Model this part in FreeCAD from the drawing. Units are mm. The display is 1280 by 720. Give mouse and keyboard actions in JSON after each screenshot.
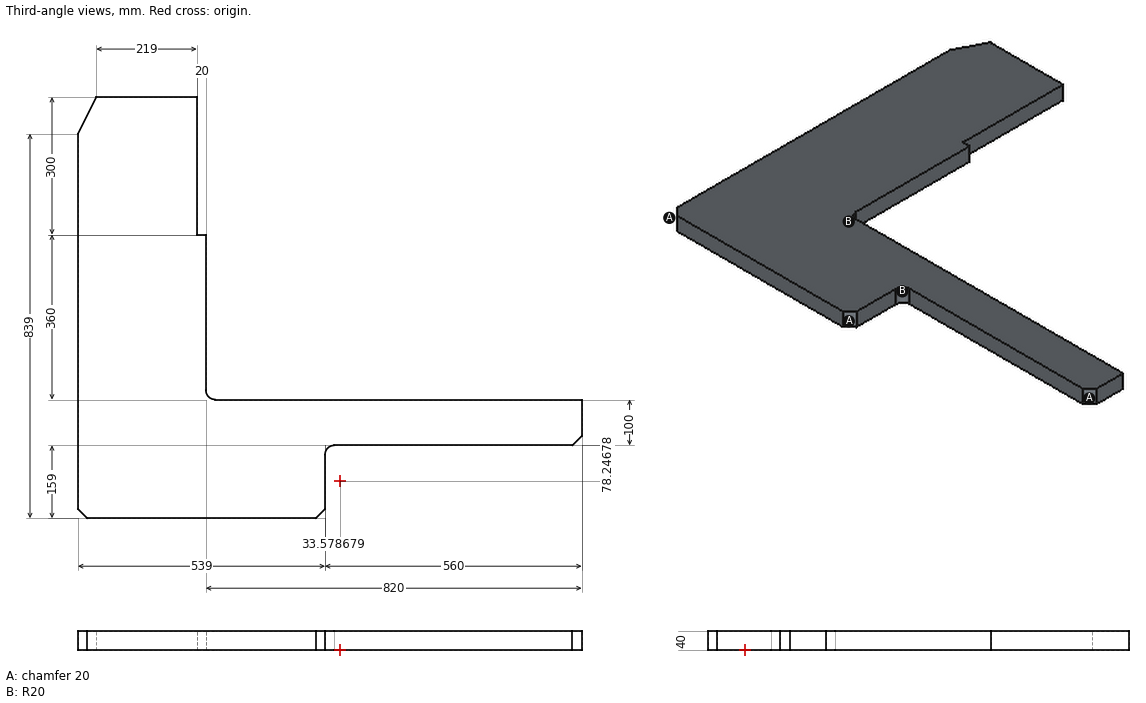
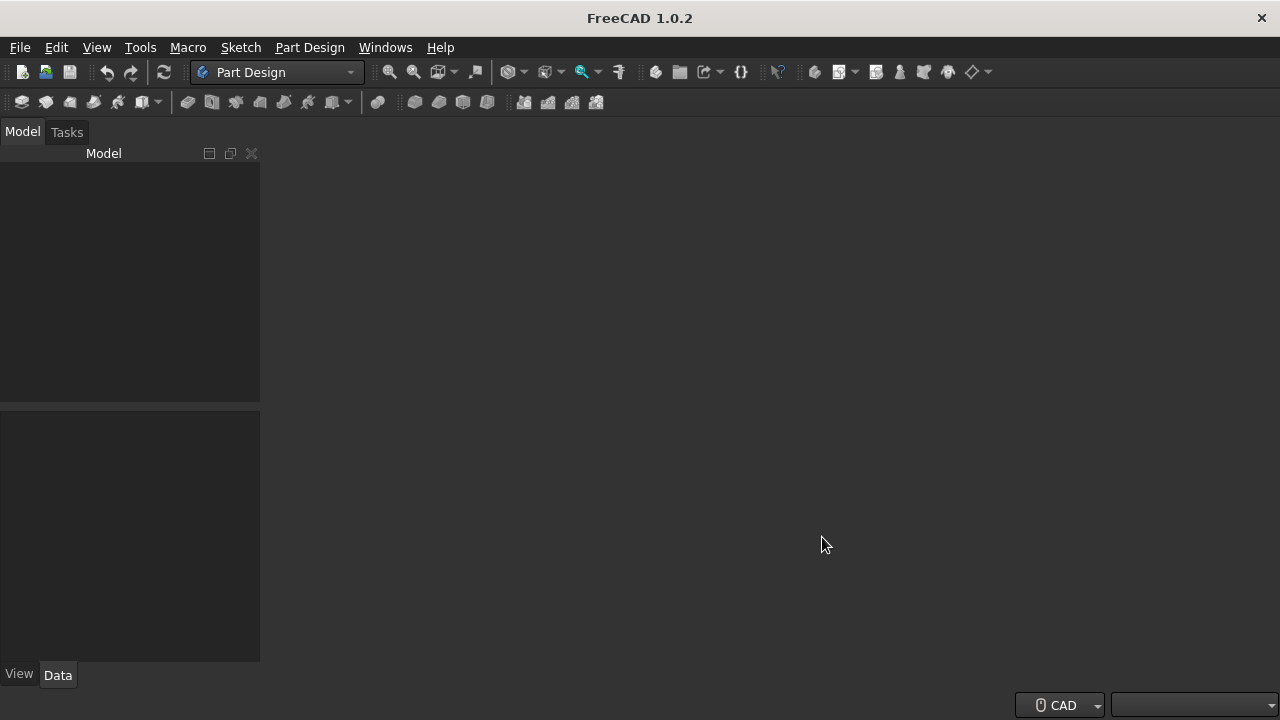
{"action": "key", "text": "ctrl+n"}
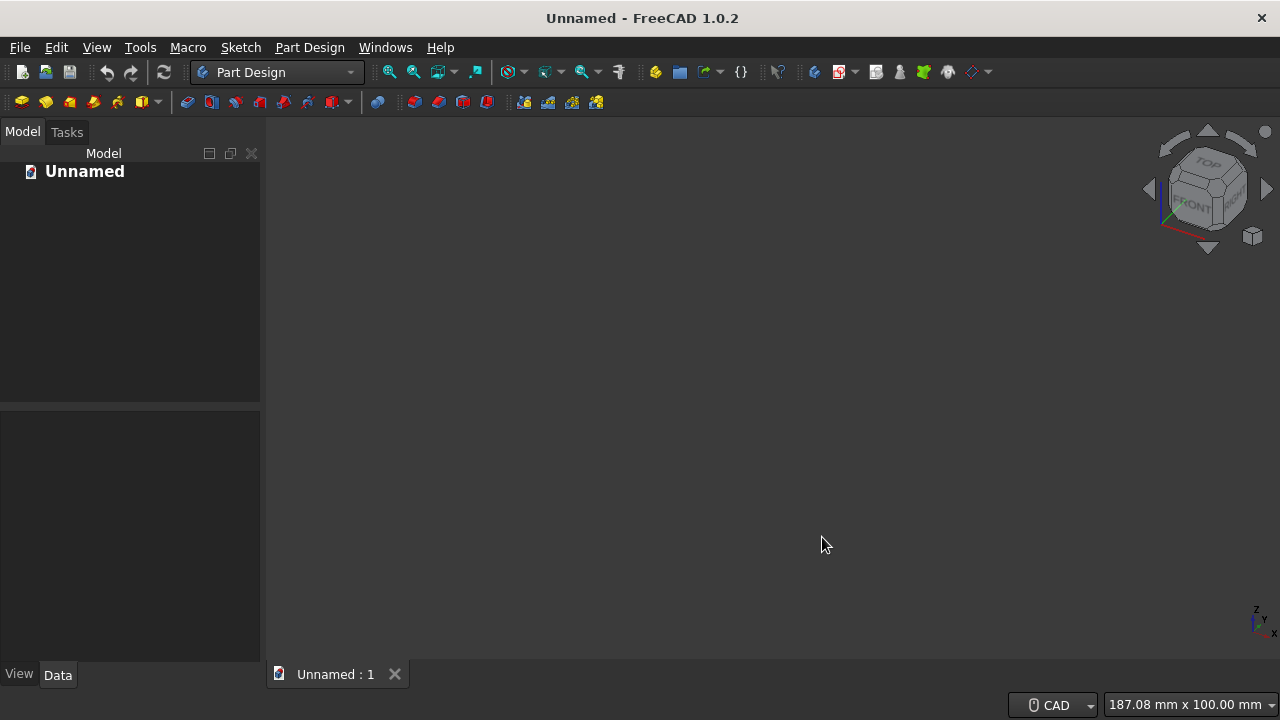
{"action": "left_click", "coordinate": [840, 72]}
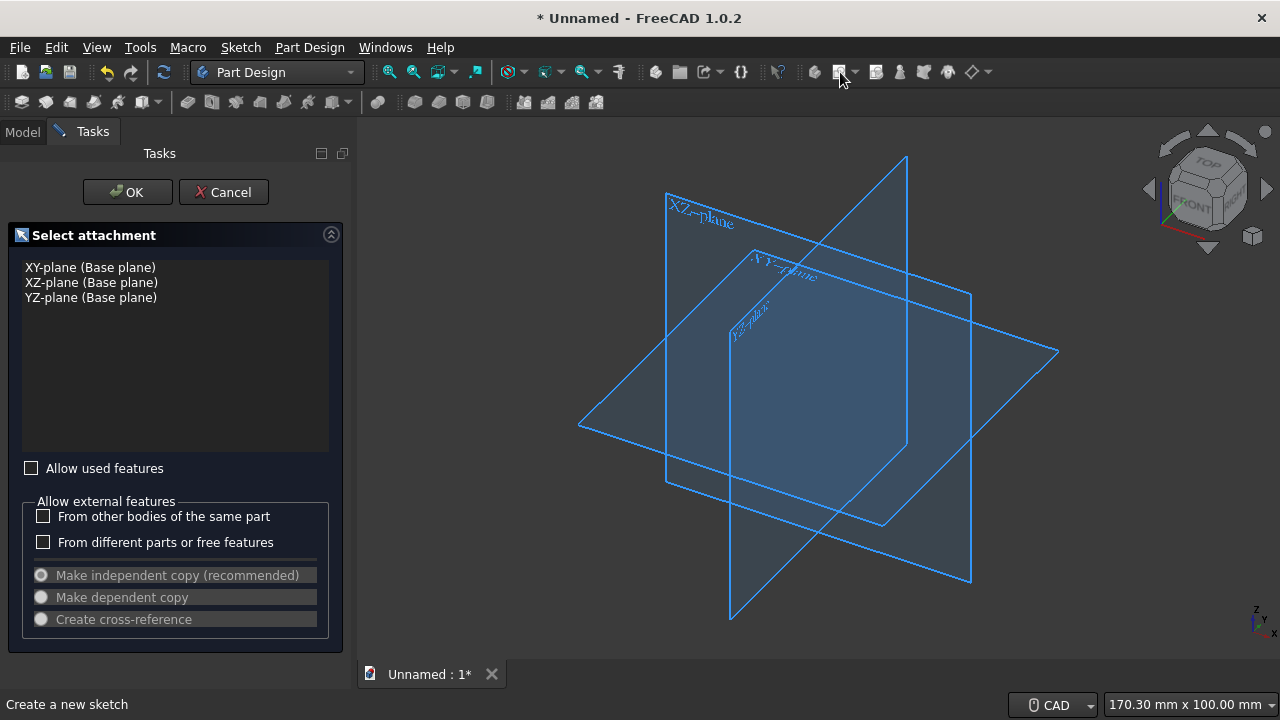
{"action": "left_click", "coordinate": [82, 268]}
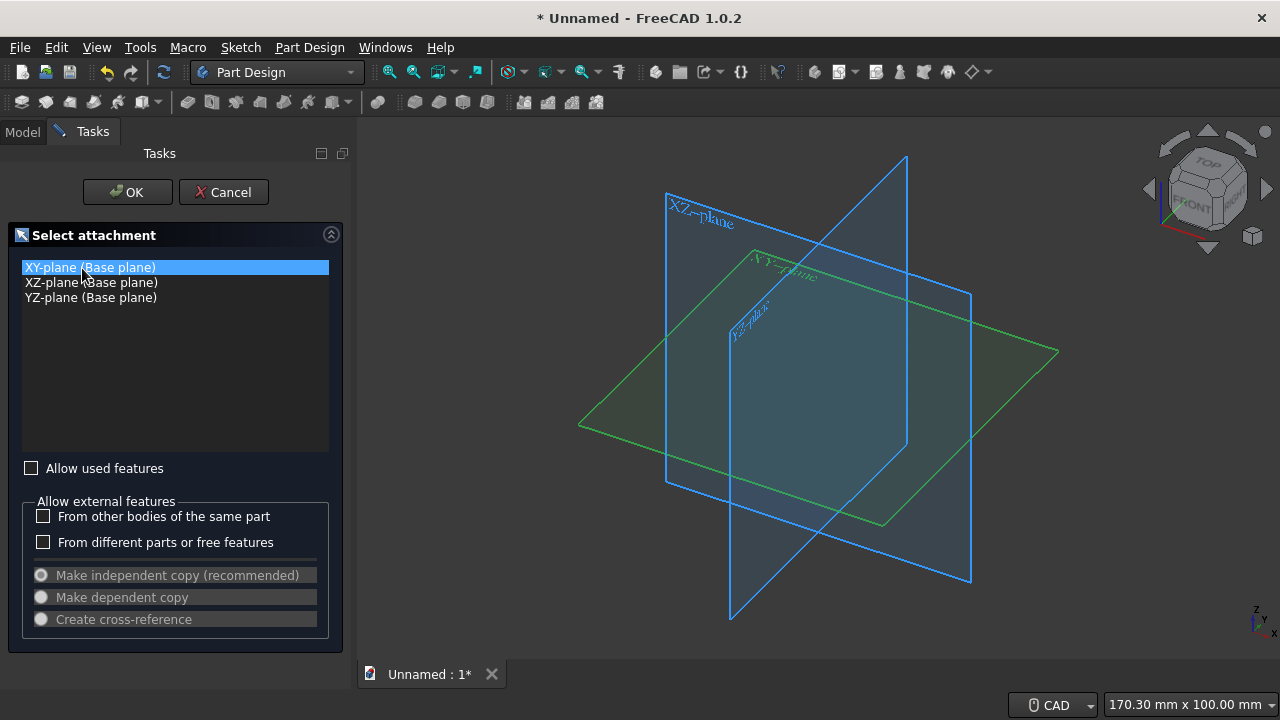
{"action": "left_click", "coordinate": [128, 192]}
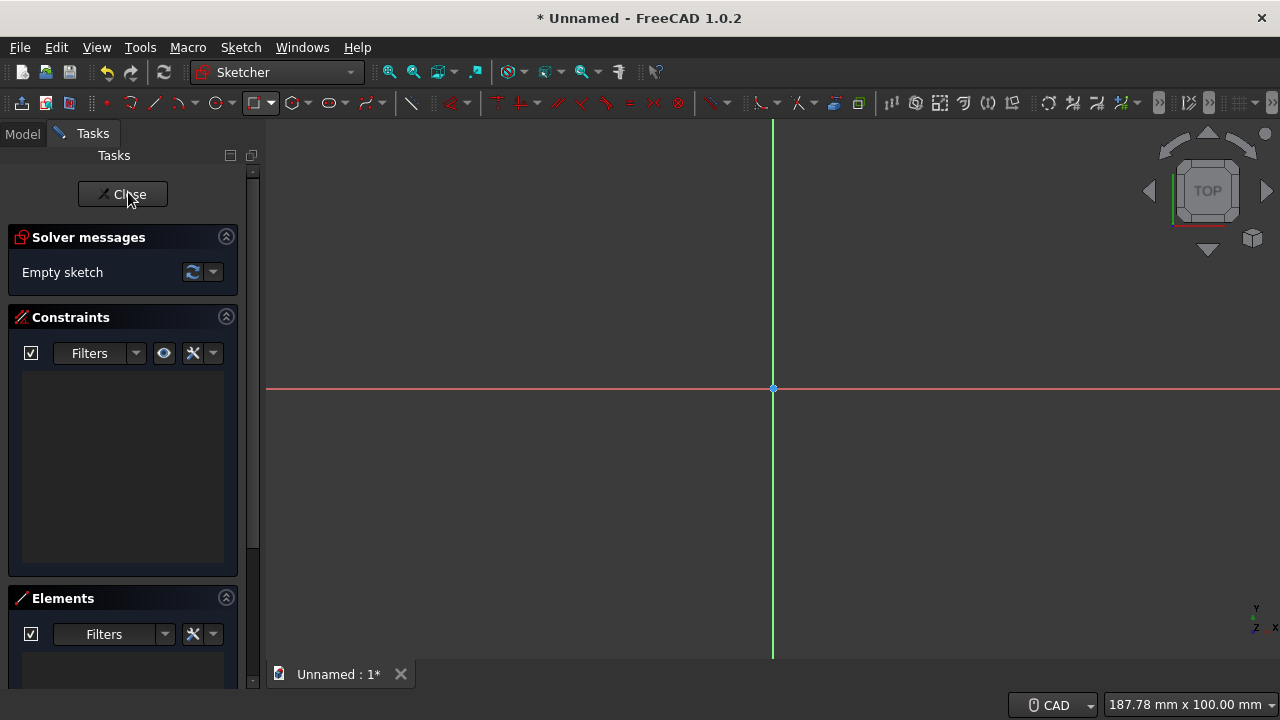
{"action": "scroll", "coordinate": [709, 553], "scroll_direction": "down", "scroll_amount": 13}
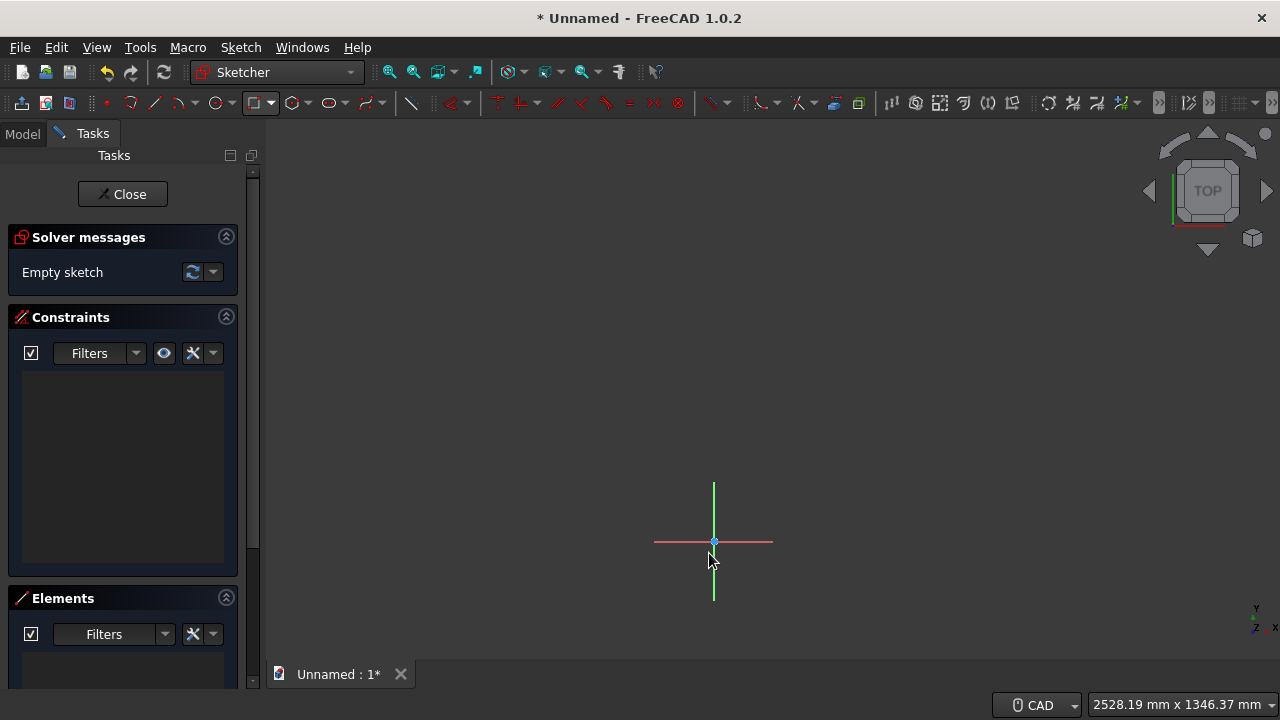
{"action": "left_click", "coordinate": [132, 104]}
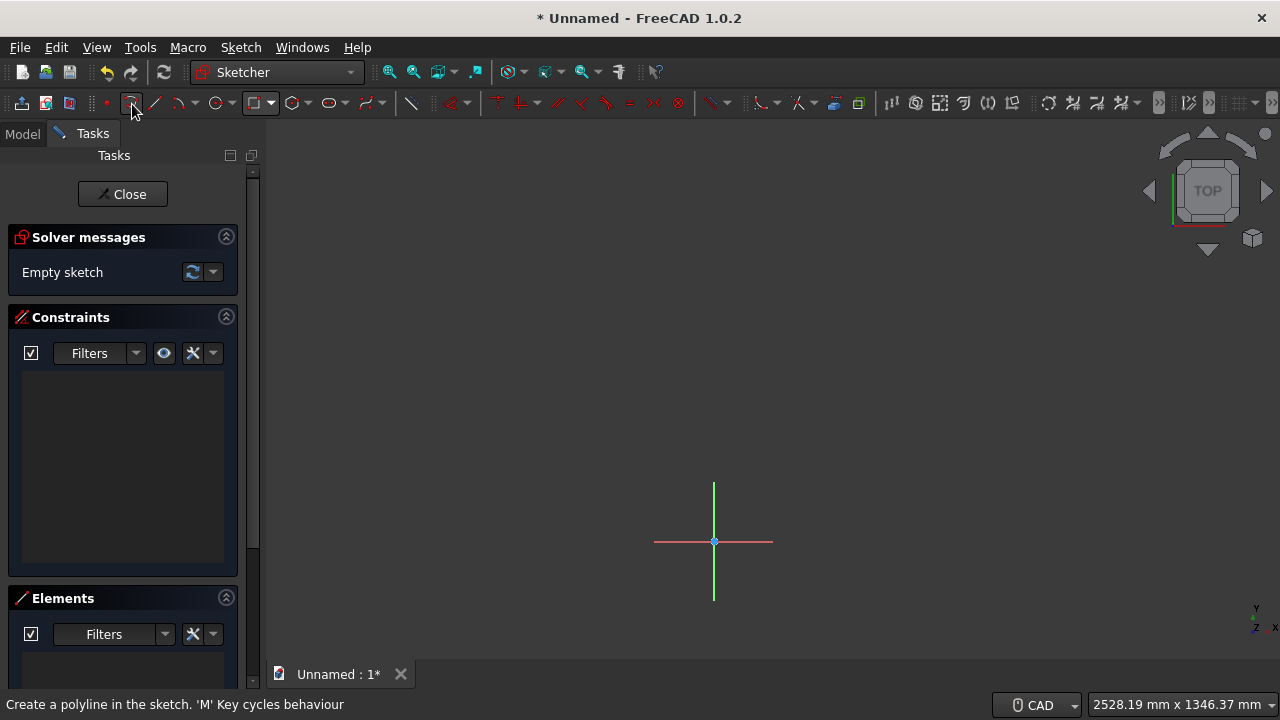
{"action": "left_click", "coordinate": [701, 510]}
{"action": "left_click", "coordinate": [925, 510]}
{"action": "left_click", "coordinate": [925, 470]}
{"action": "left_click", "coordinate": [596, 470]}
{"action": "left_click", "coordinate": [596, 326]}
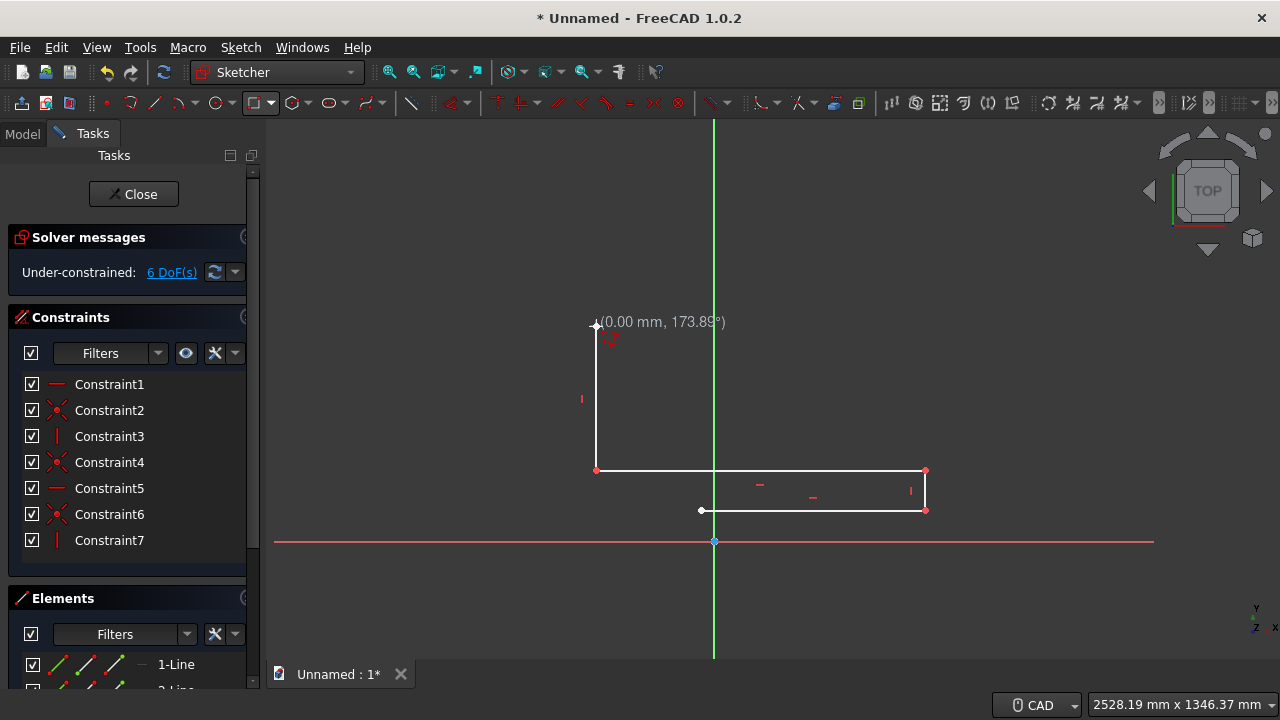
{"action": "scroll", "coordinate": [588, 326], "scroll_direction": "up", "scroll_amount": 4}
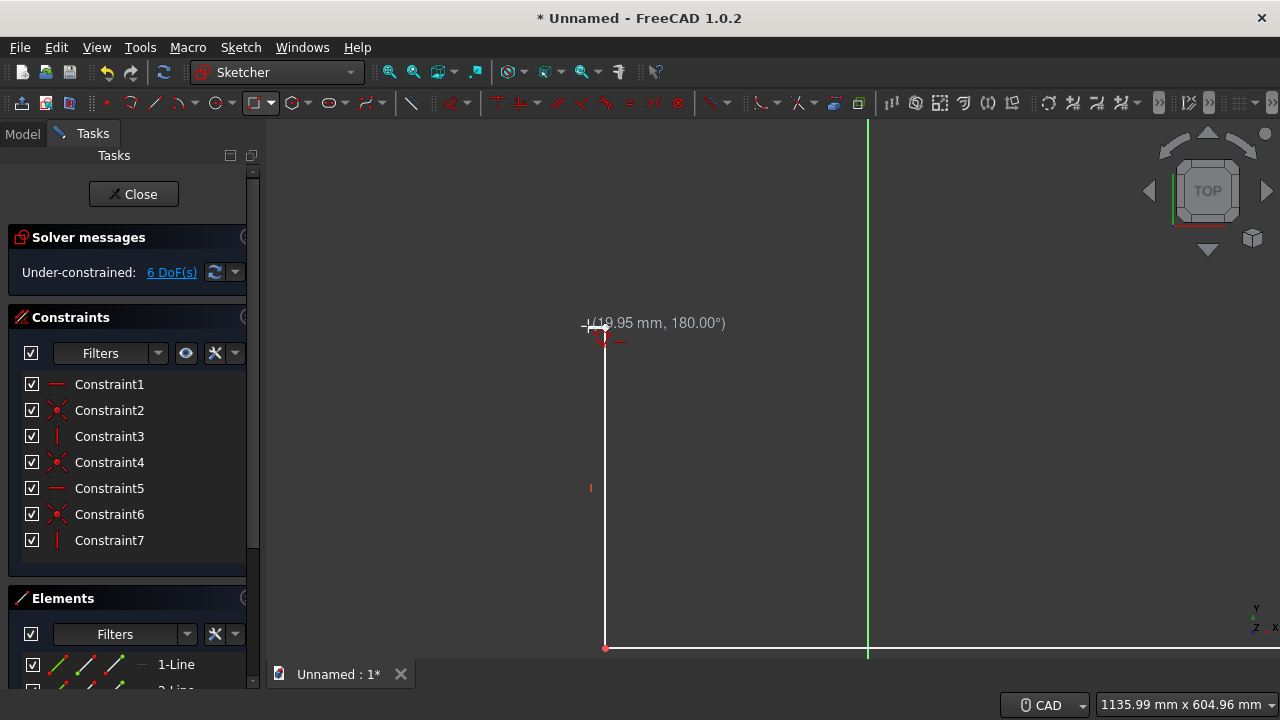
{"action": "left_click", "coordinate": [588, 326]}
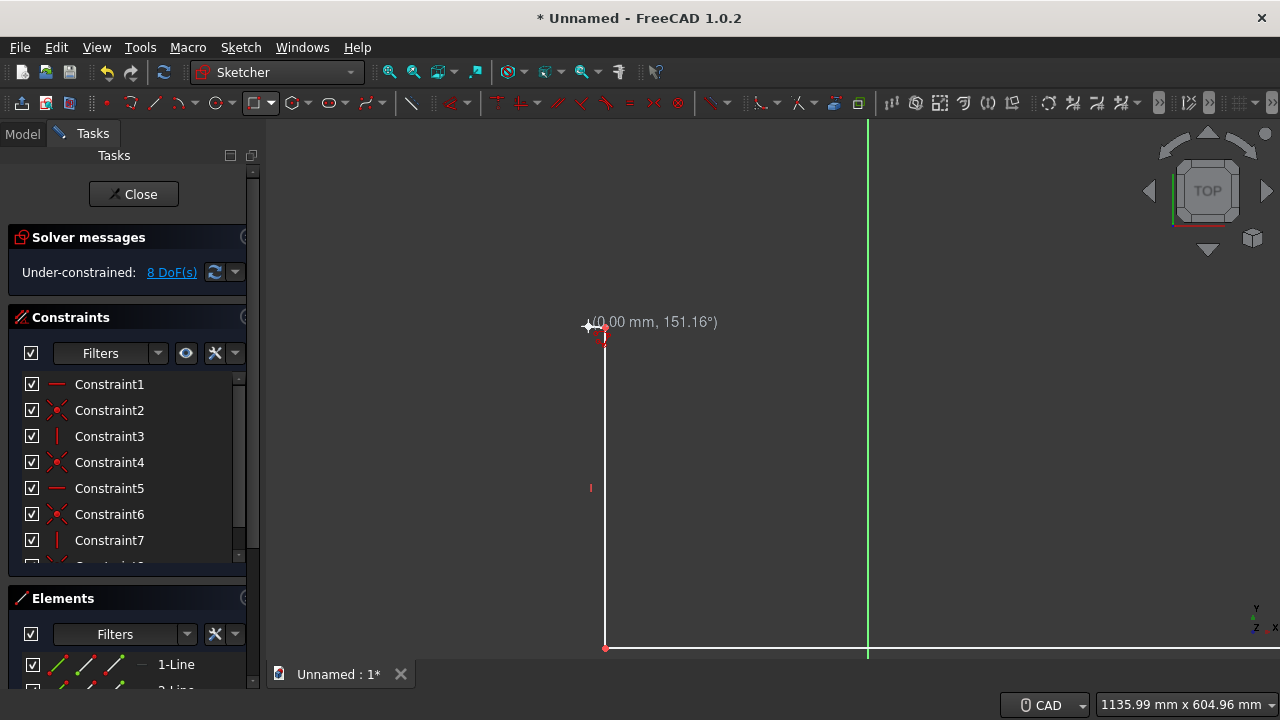
{"action": "scroll", "coordinate": [588, 325], "scroll_direction": "down", "scroll_amount": 4}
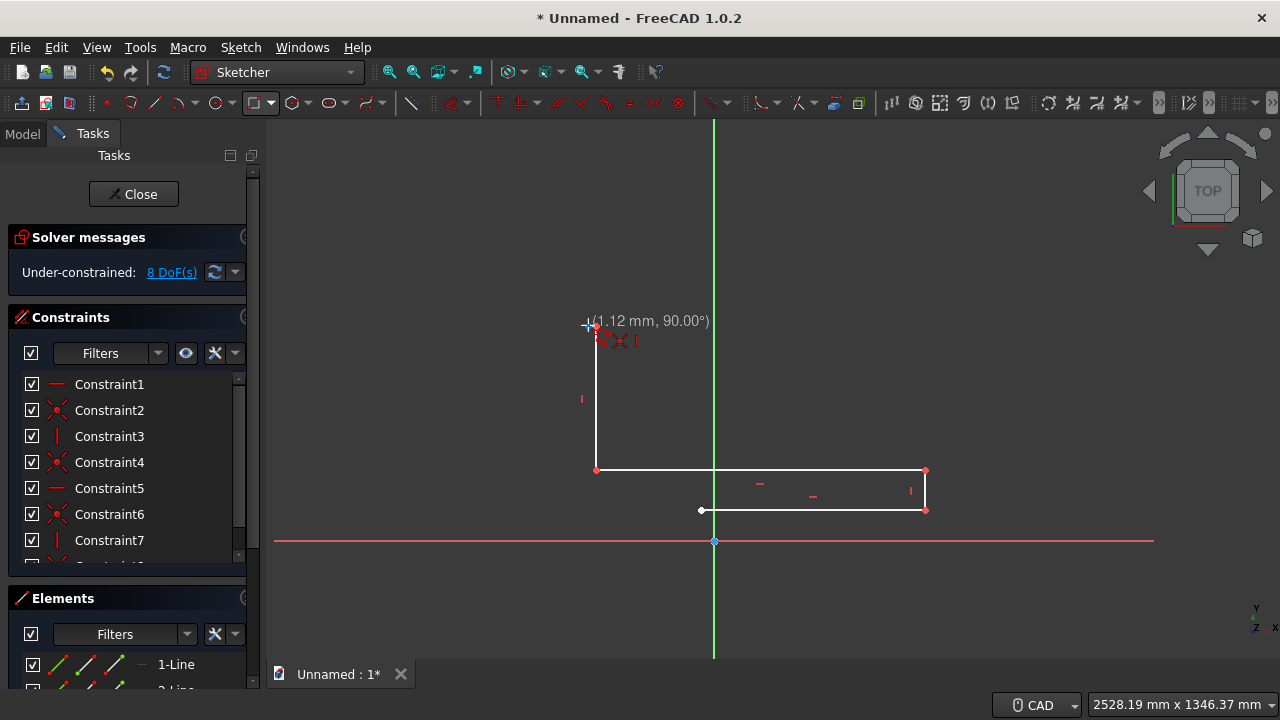
{"action": "left_click", "coordinate": [588, 205]}
{"action": "left_click", "coordinate": [501, 205]}
{"action": "left_click", "coordinate": [485, 237]}
{"action": "left_click", "coordinate": [485, 573]}
{"action": "left_click", "coordinate": [701, 573]}
{"action": "left_click", "coordinate": [701, 510]}
{"action": "key", "text": "Escape"}
{"action": "key", "text": "Escape"}